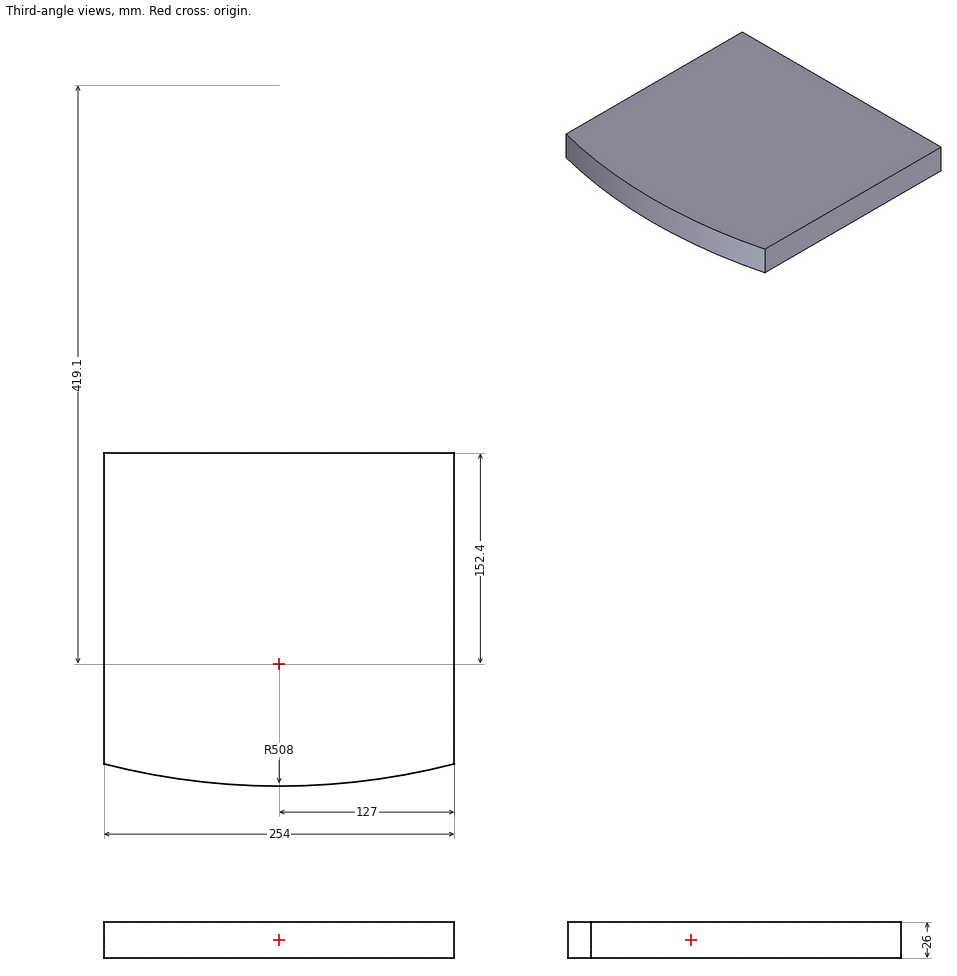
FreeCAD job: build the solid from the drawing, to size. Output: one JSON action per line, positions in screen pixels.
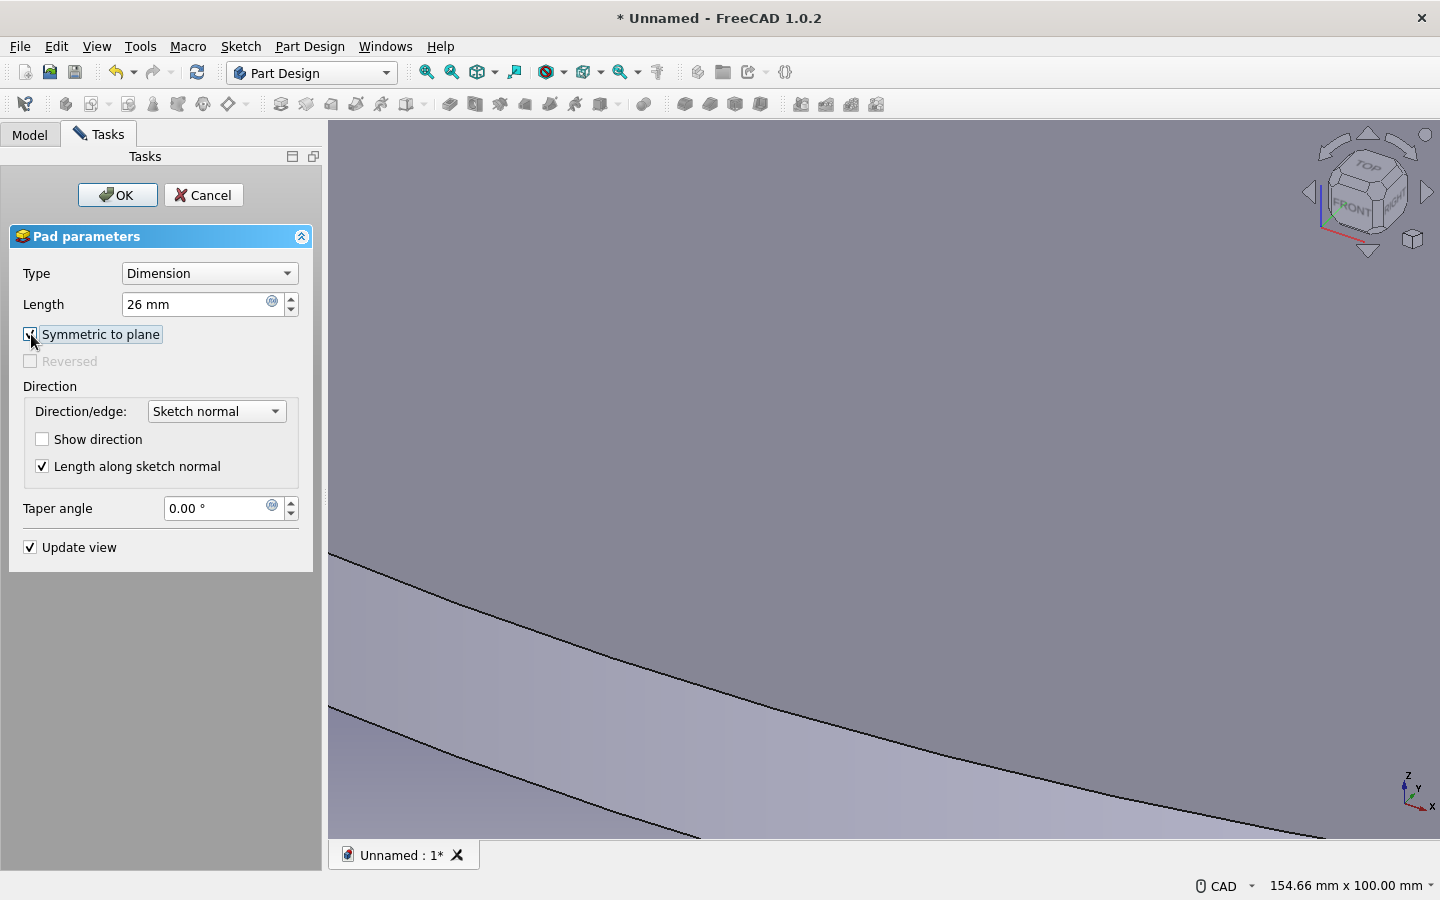
{"action": "left_click", "coordinate": [118, 195]}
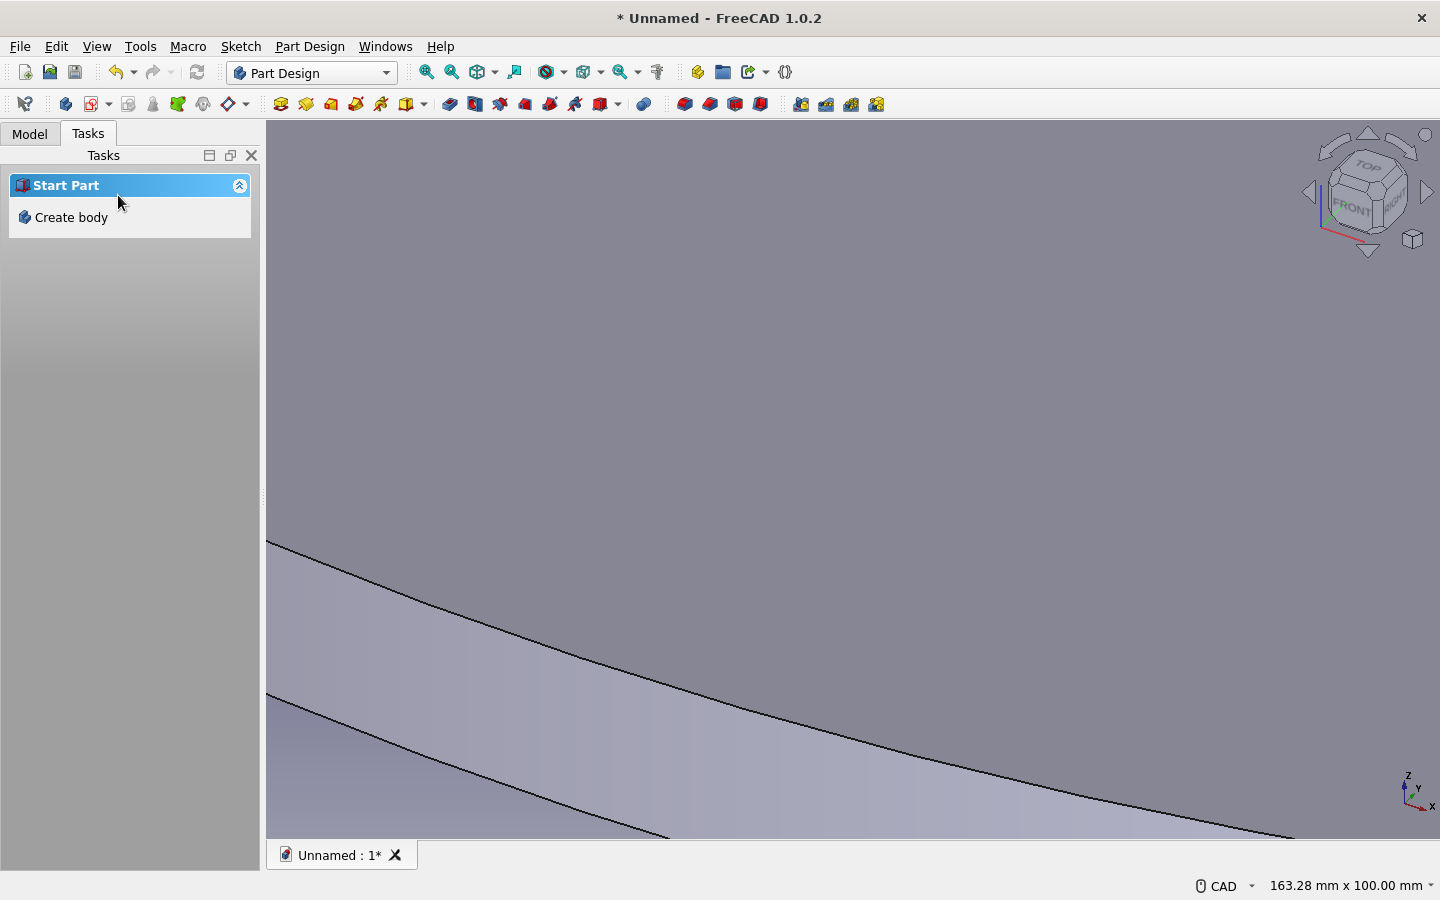
{"action": "key", "text": "0"}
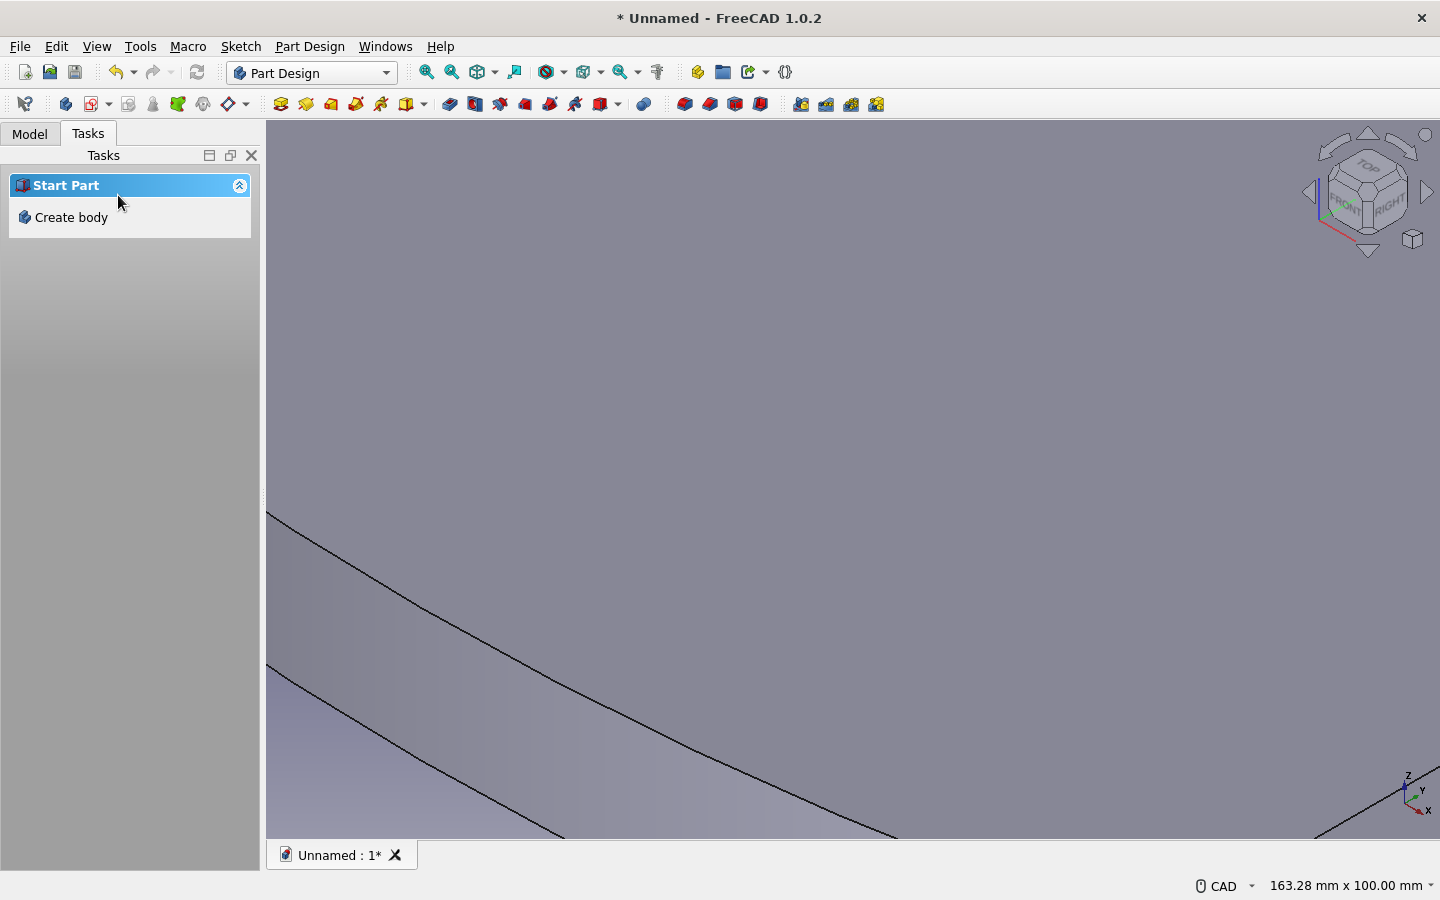
{"action": "left_click", "coordinate": [427, 72]}